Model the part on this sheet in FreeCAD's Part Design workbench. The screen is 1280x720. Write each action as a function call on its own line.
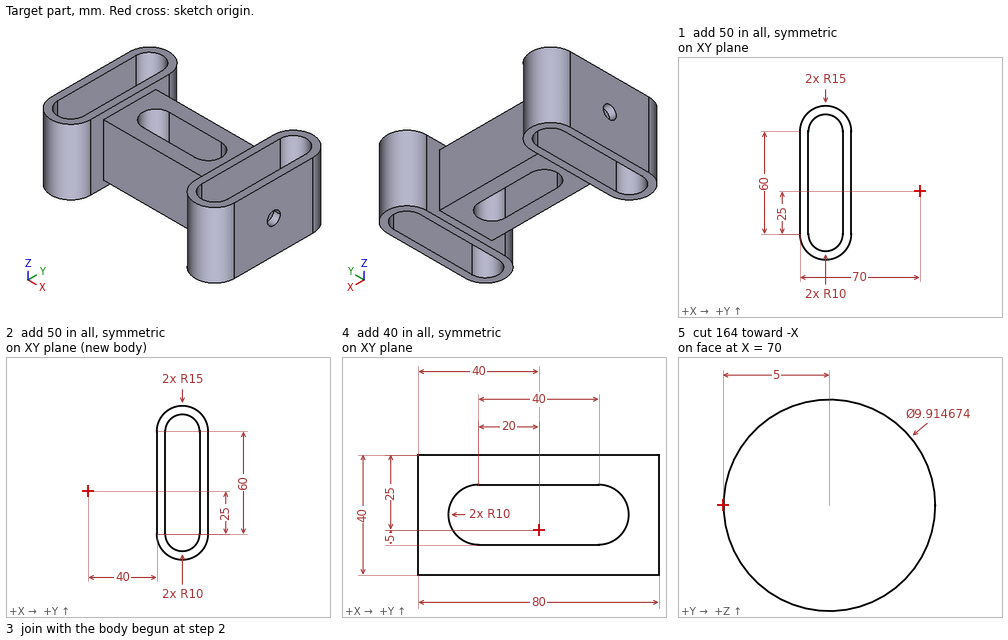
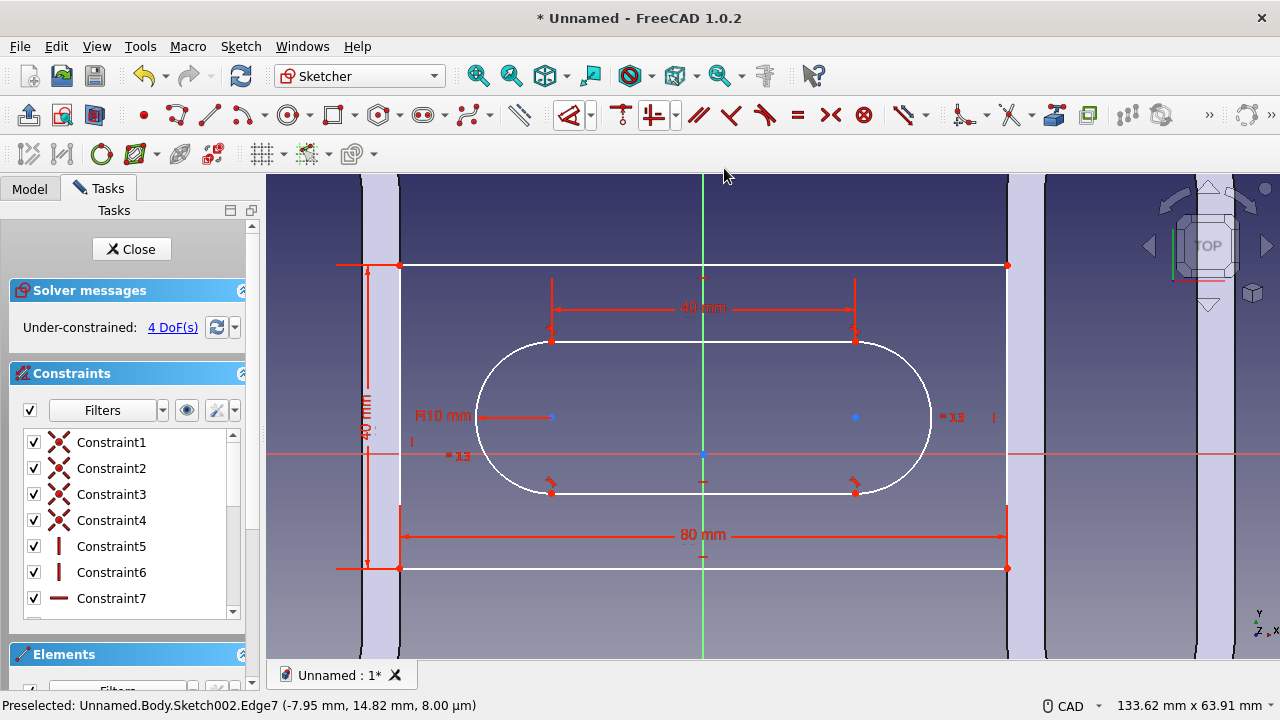
click(552, 494)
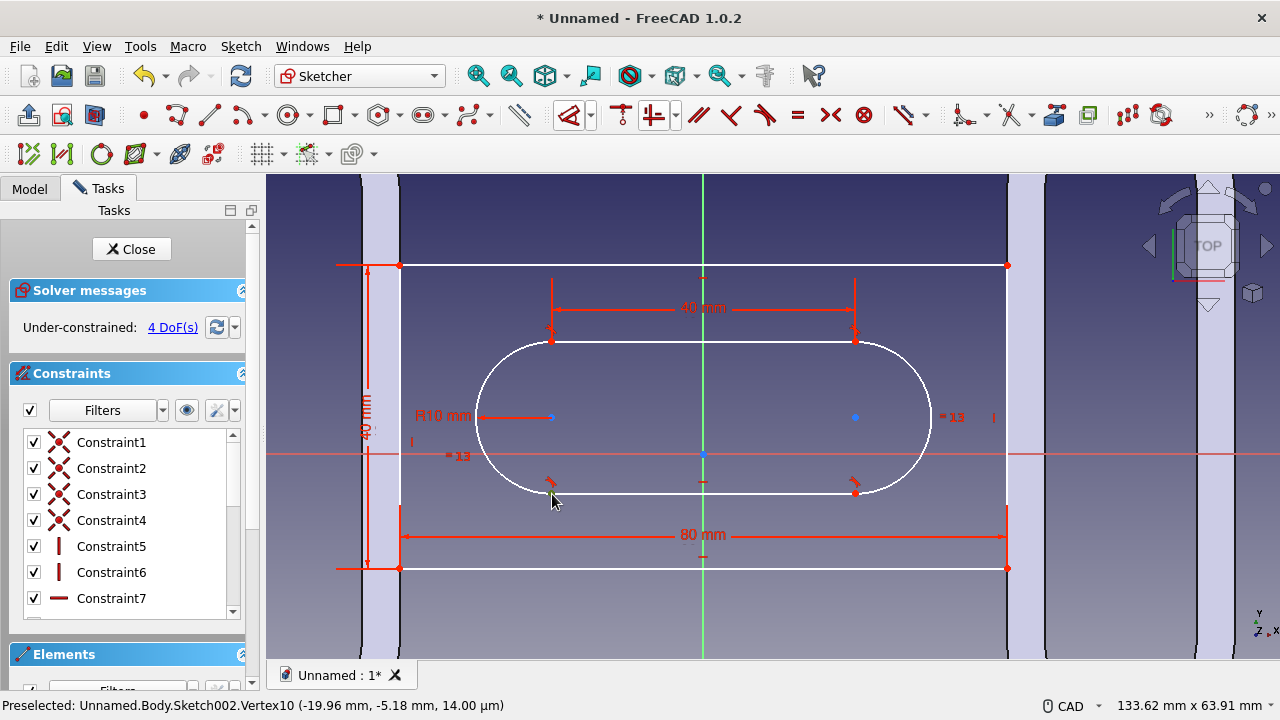
click(590, 116)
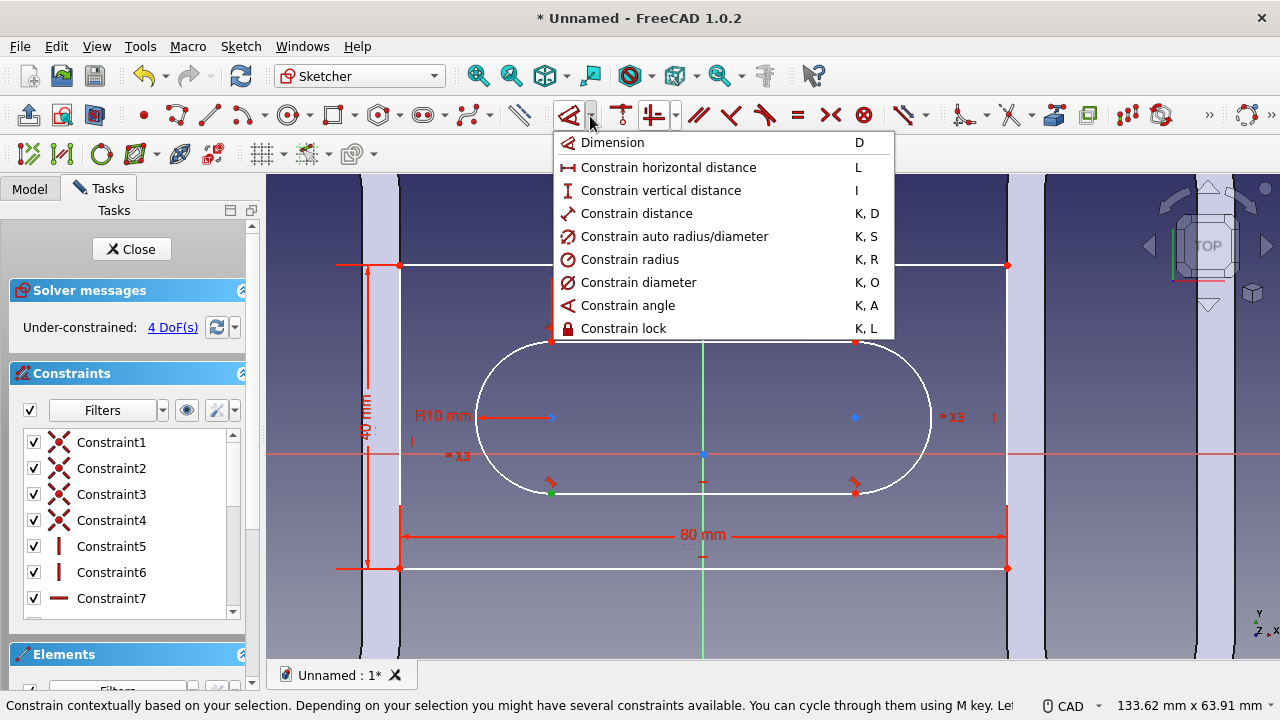
click(724, 190)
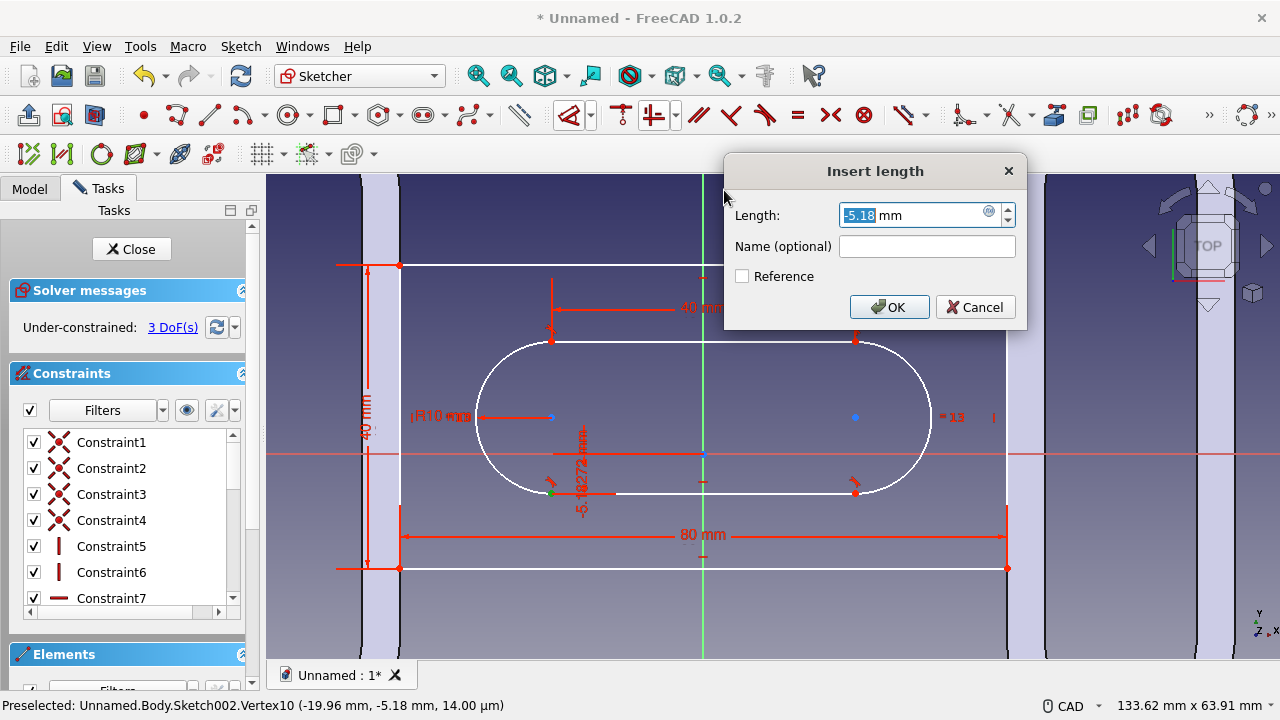
text(-5)
key(Return)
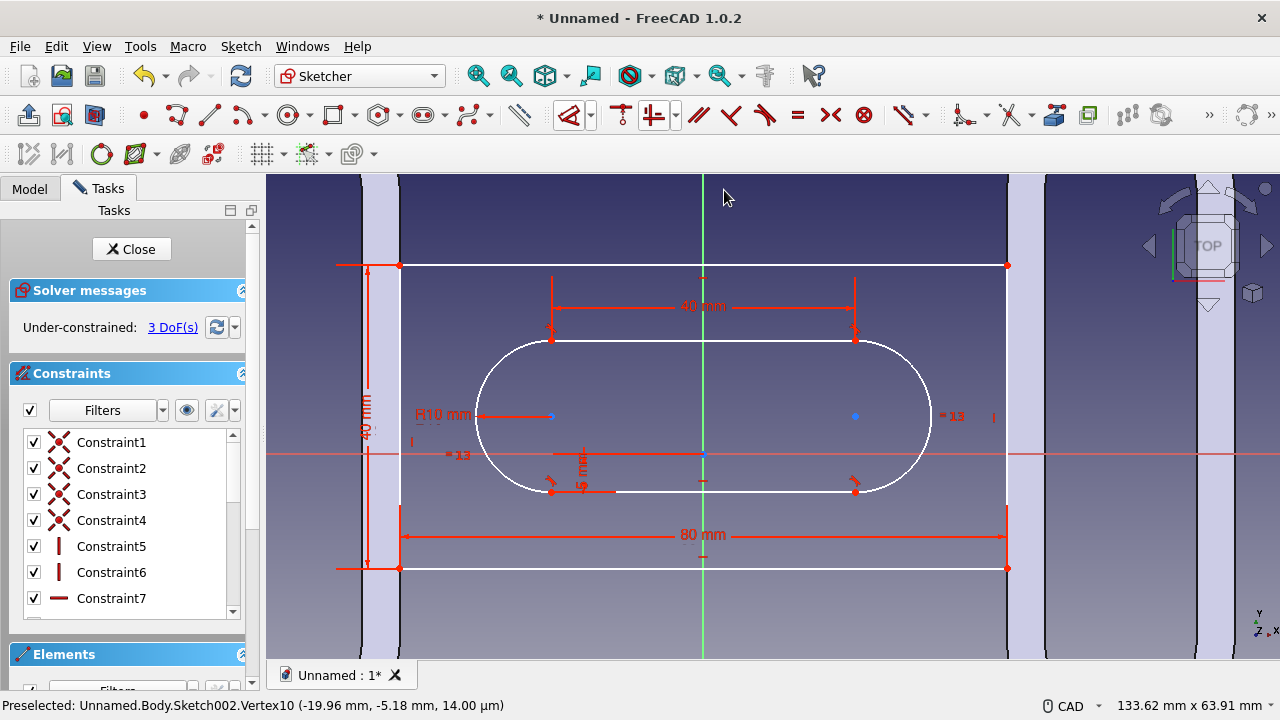
click(400, 265)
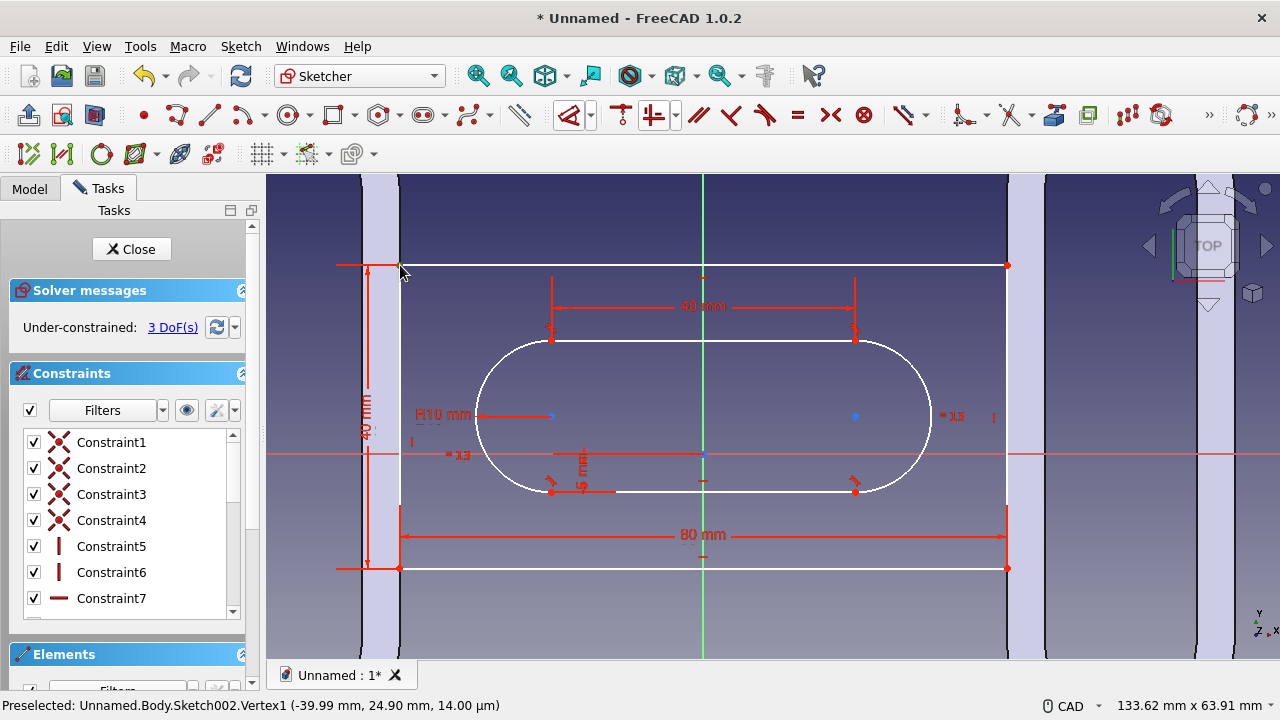
click(590, 116)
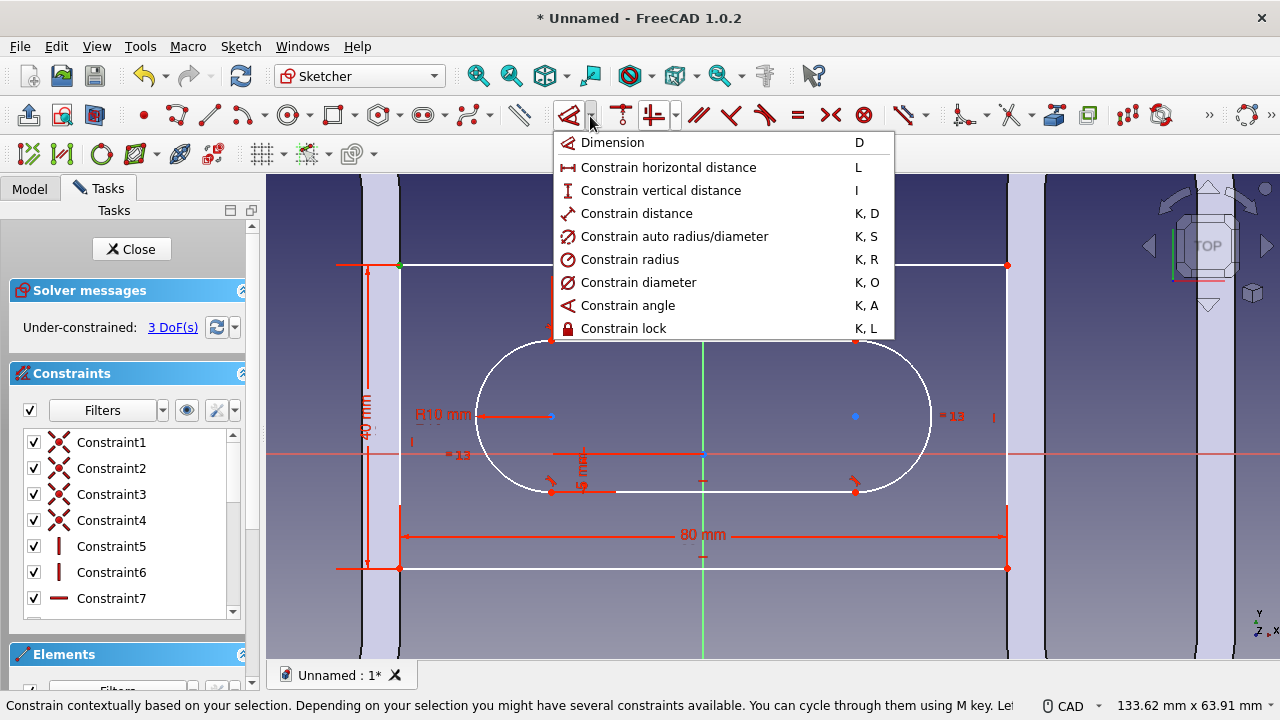
click(724, 168)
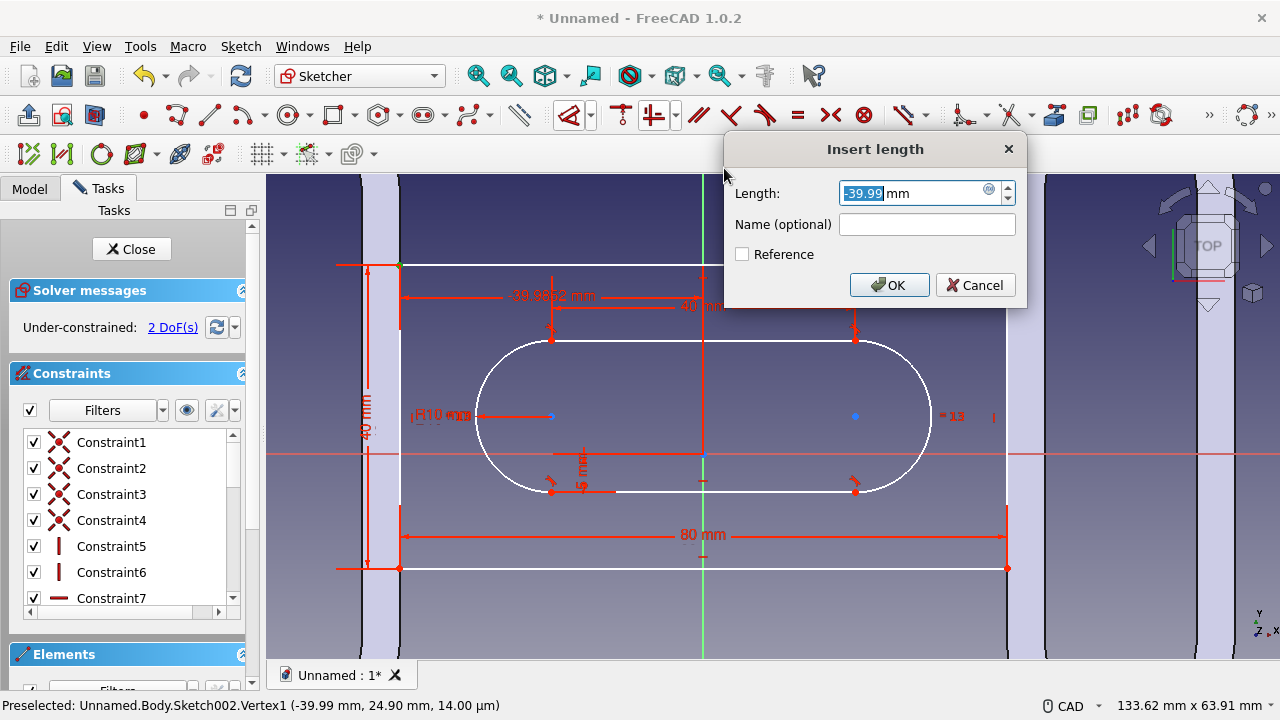
text(-40)
key(Return)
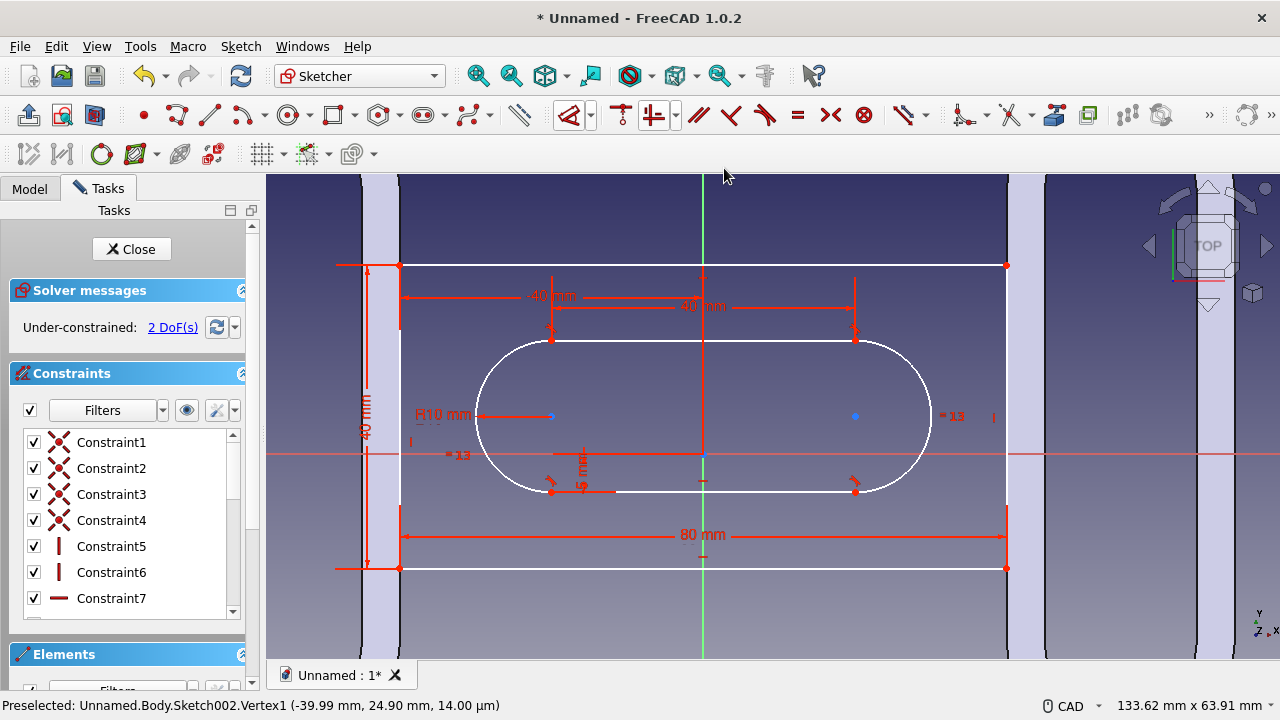
click(400, 265)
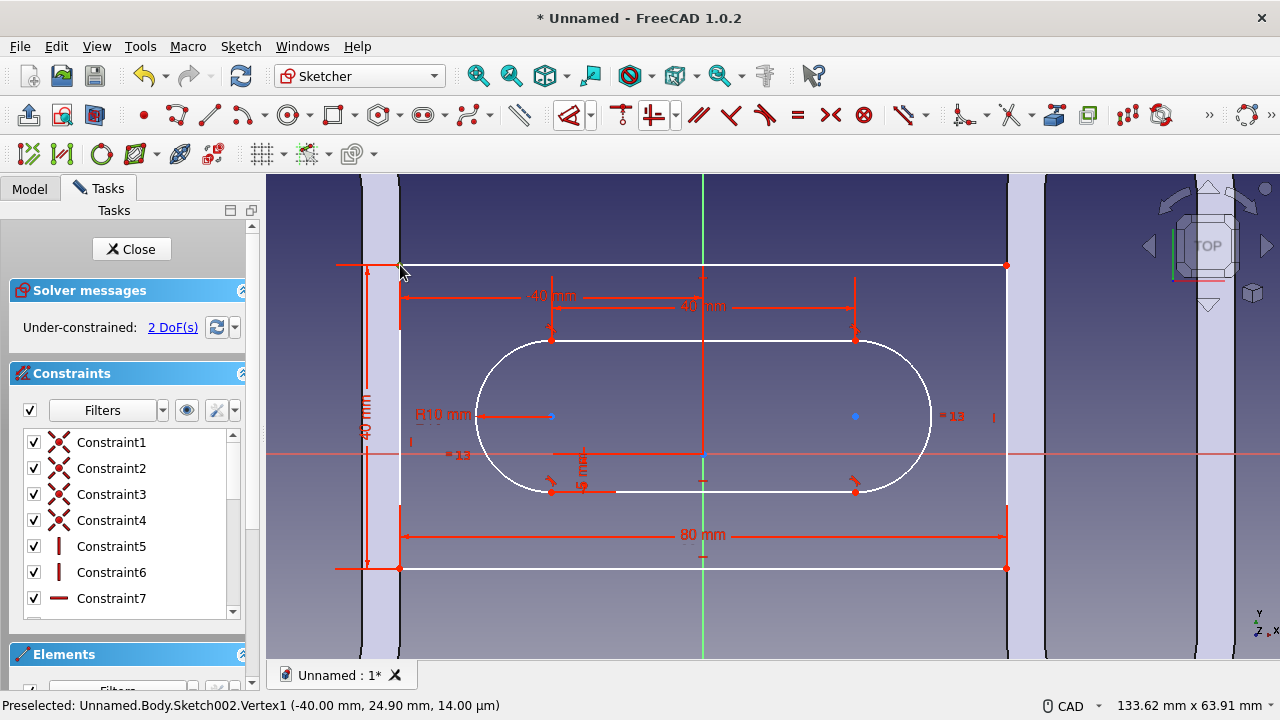
key(i)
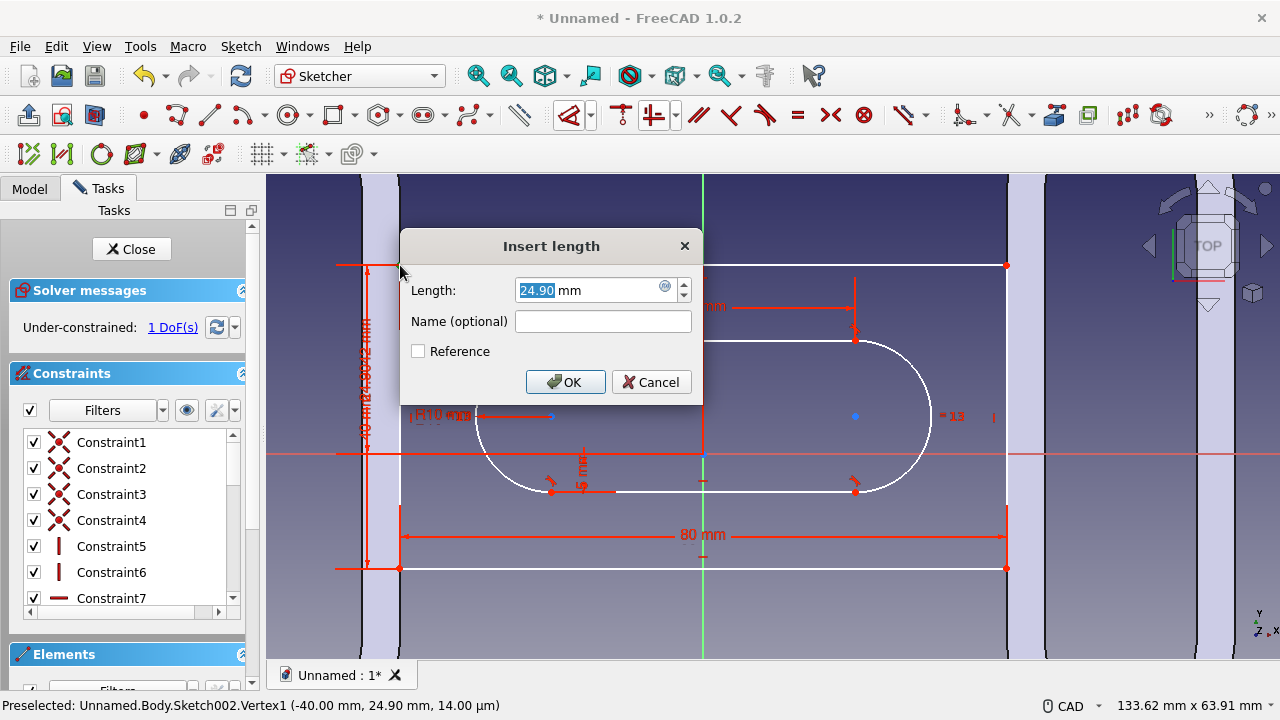
text(25)
key(Return)